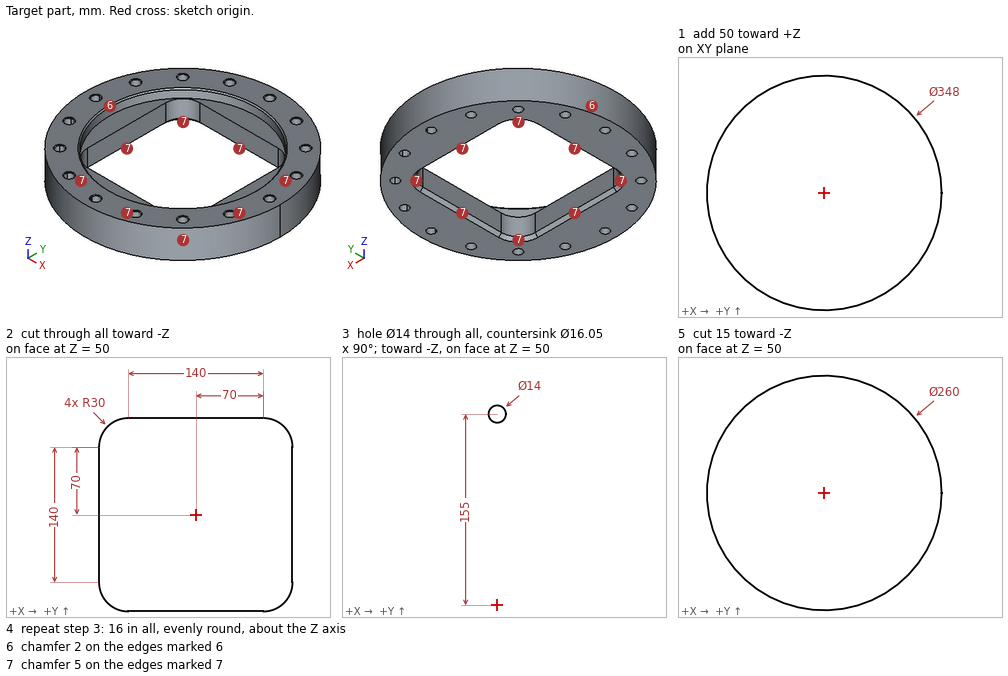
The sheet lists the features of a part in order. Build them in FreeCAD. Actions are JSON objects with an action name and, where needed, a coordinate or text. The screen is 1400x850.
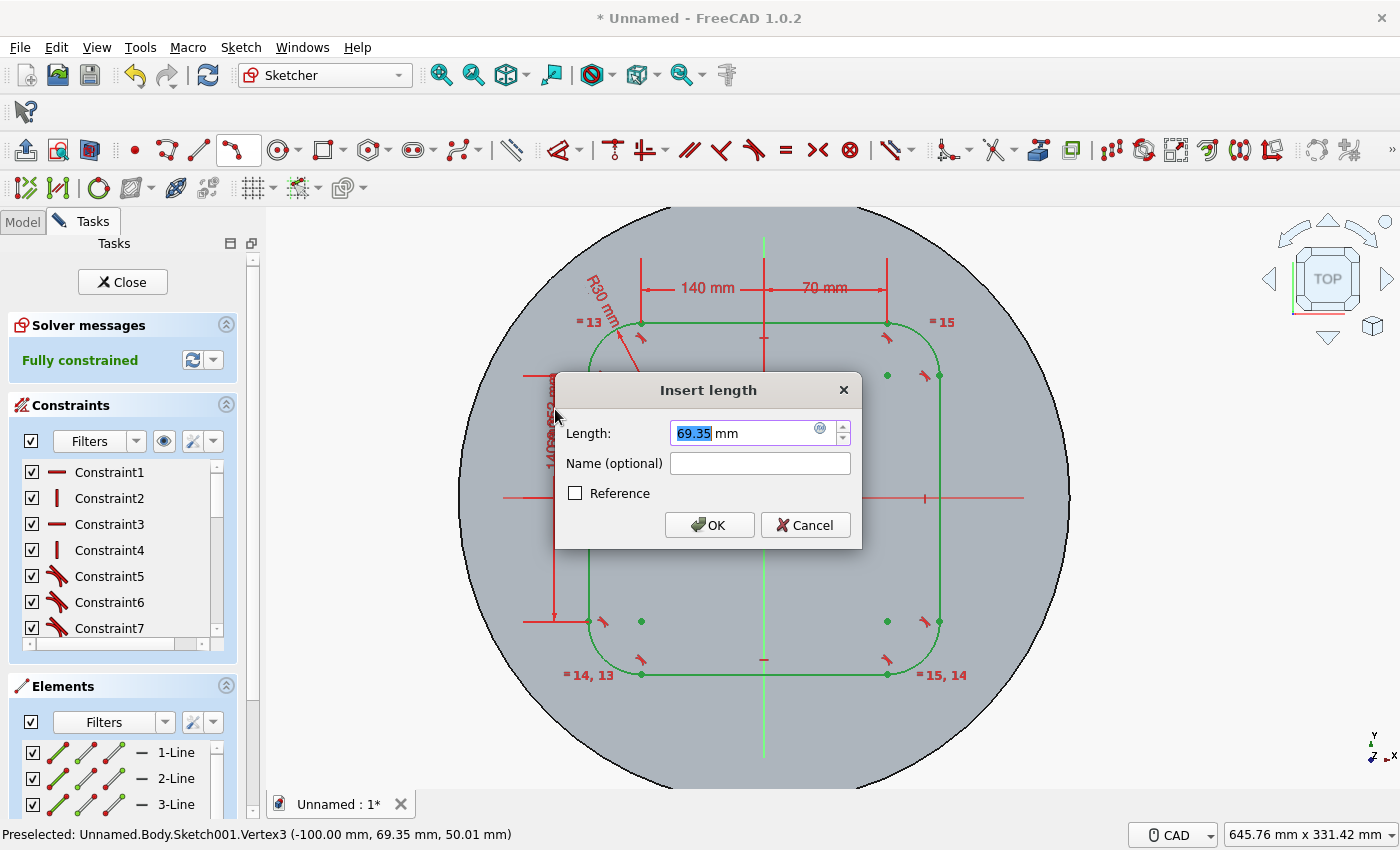
{"action": "type", "text": "70"}
{"action": "key", "text": "Return"}
{"action": "key", "text": "Escape"}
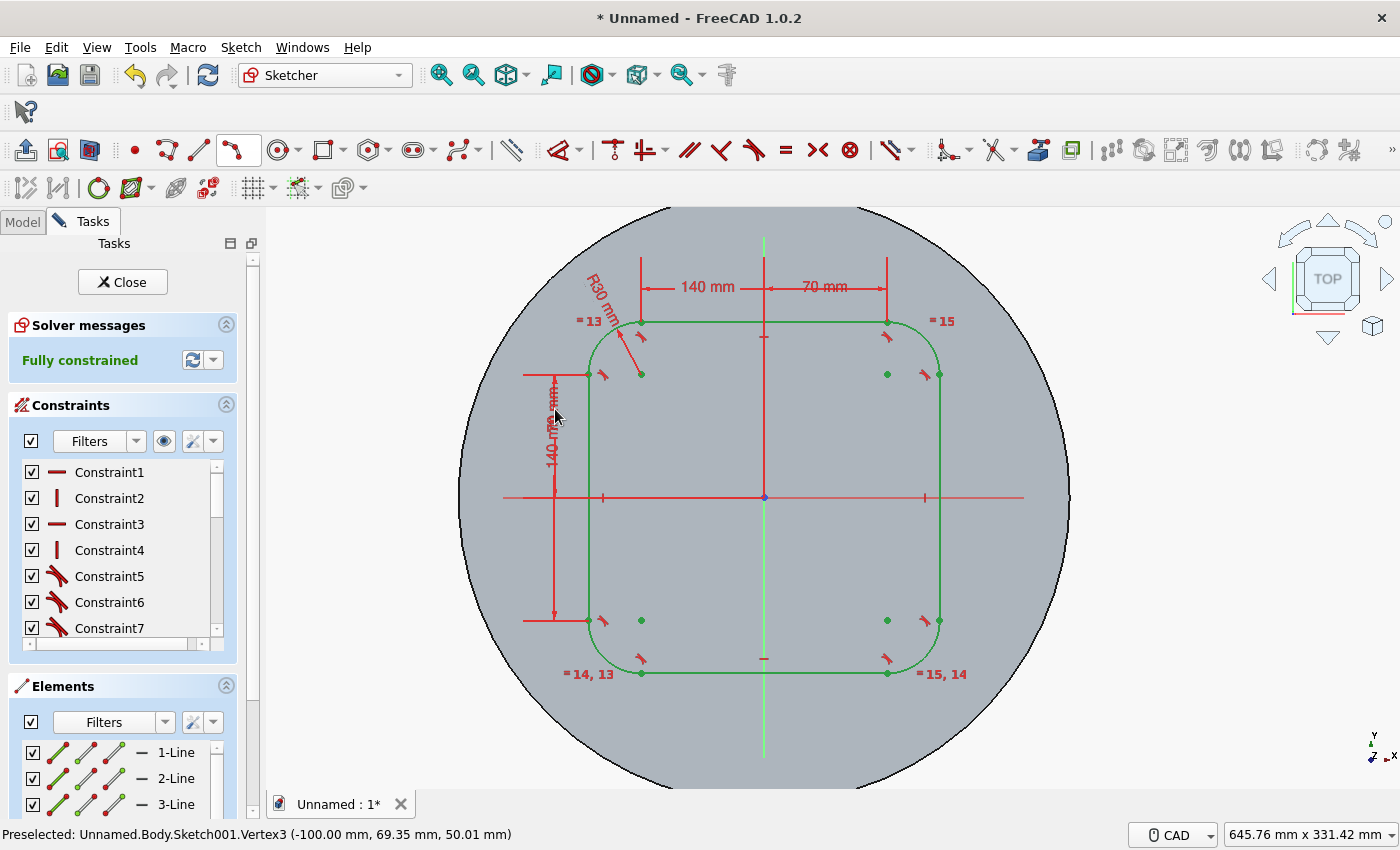
{"action": "left_click", "coordinate": [123, 282]}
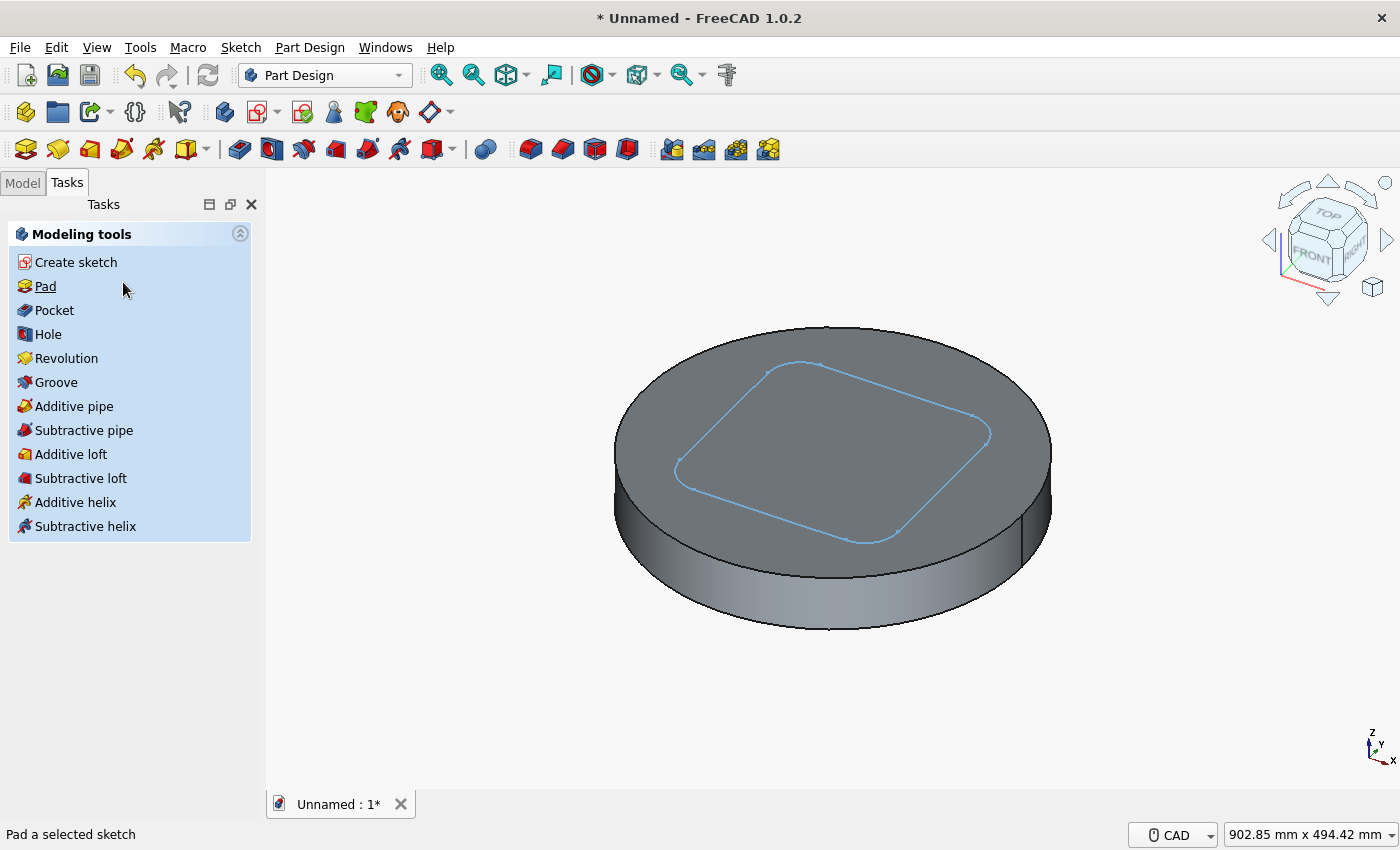
{"action": "left_click", "coordinate": [240, 150]}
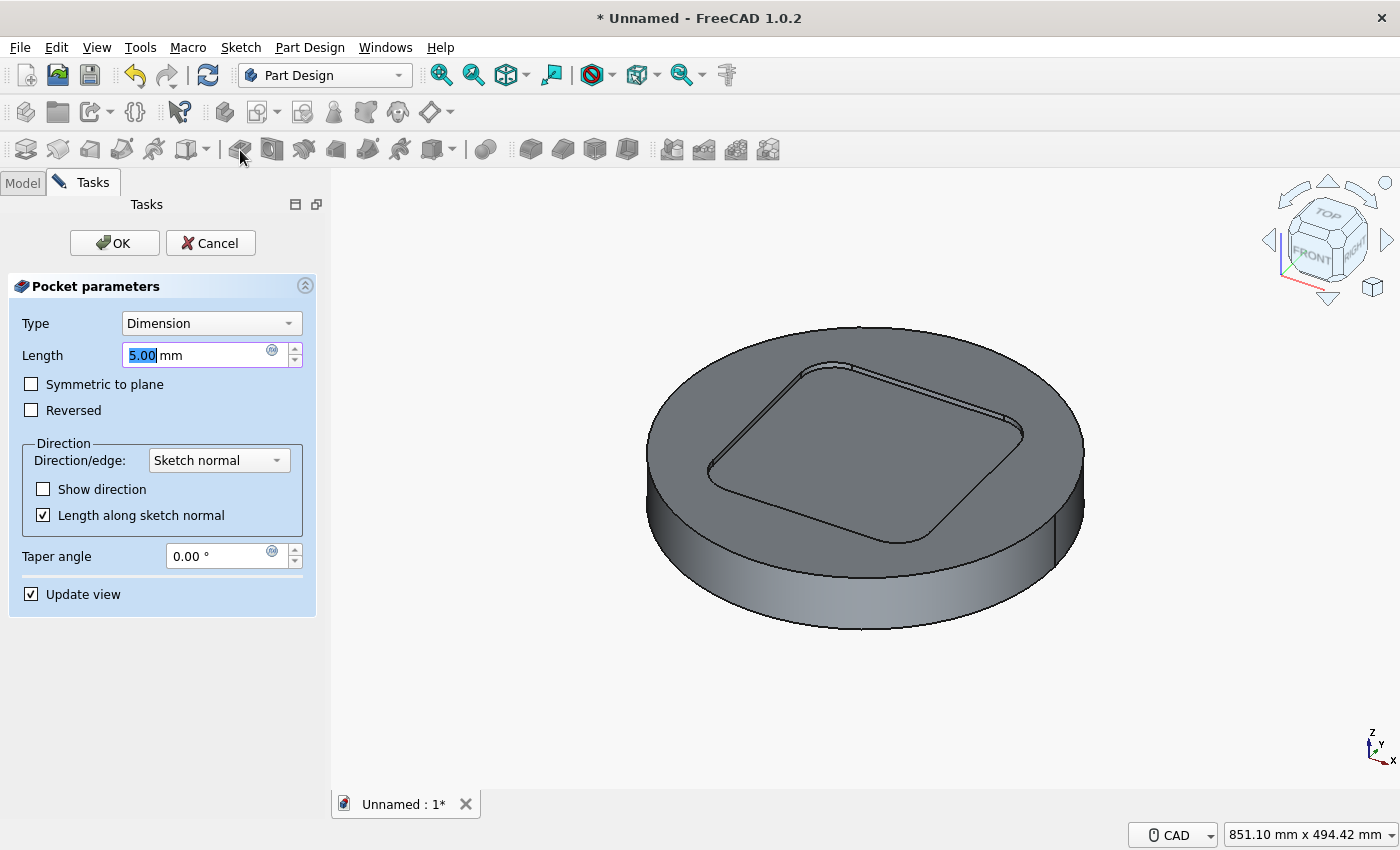
{"action": "left_click", "coordinate": [212, 324]}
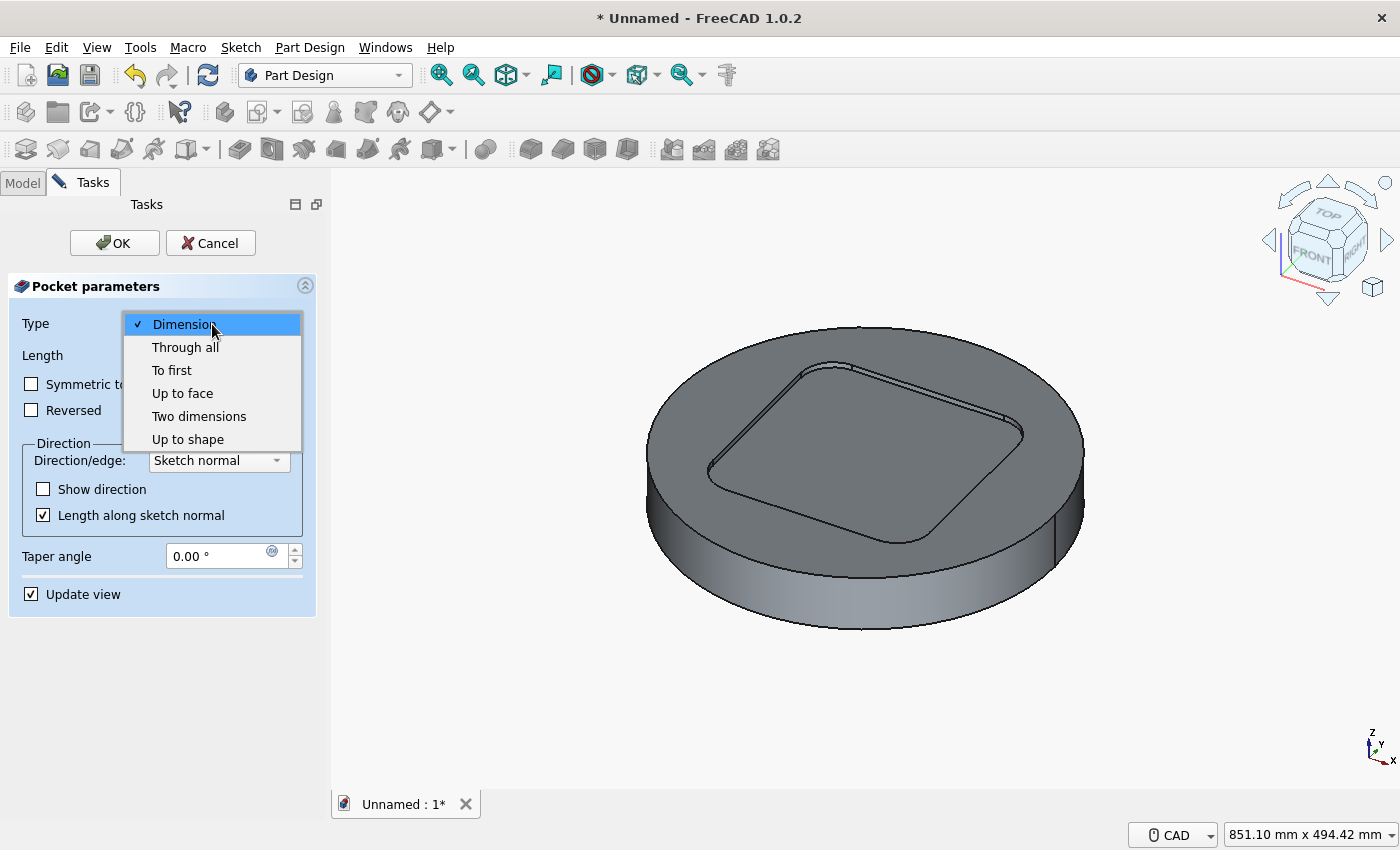
{"action": "left_click", "coordinate": [212, 348]}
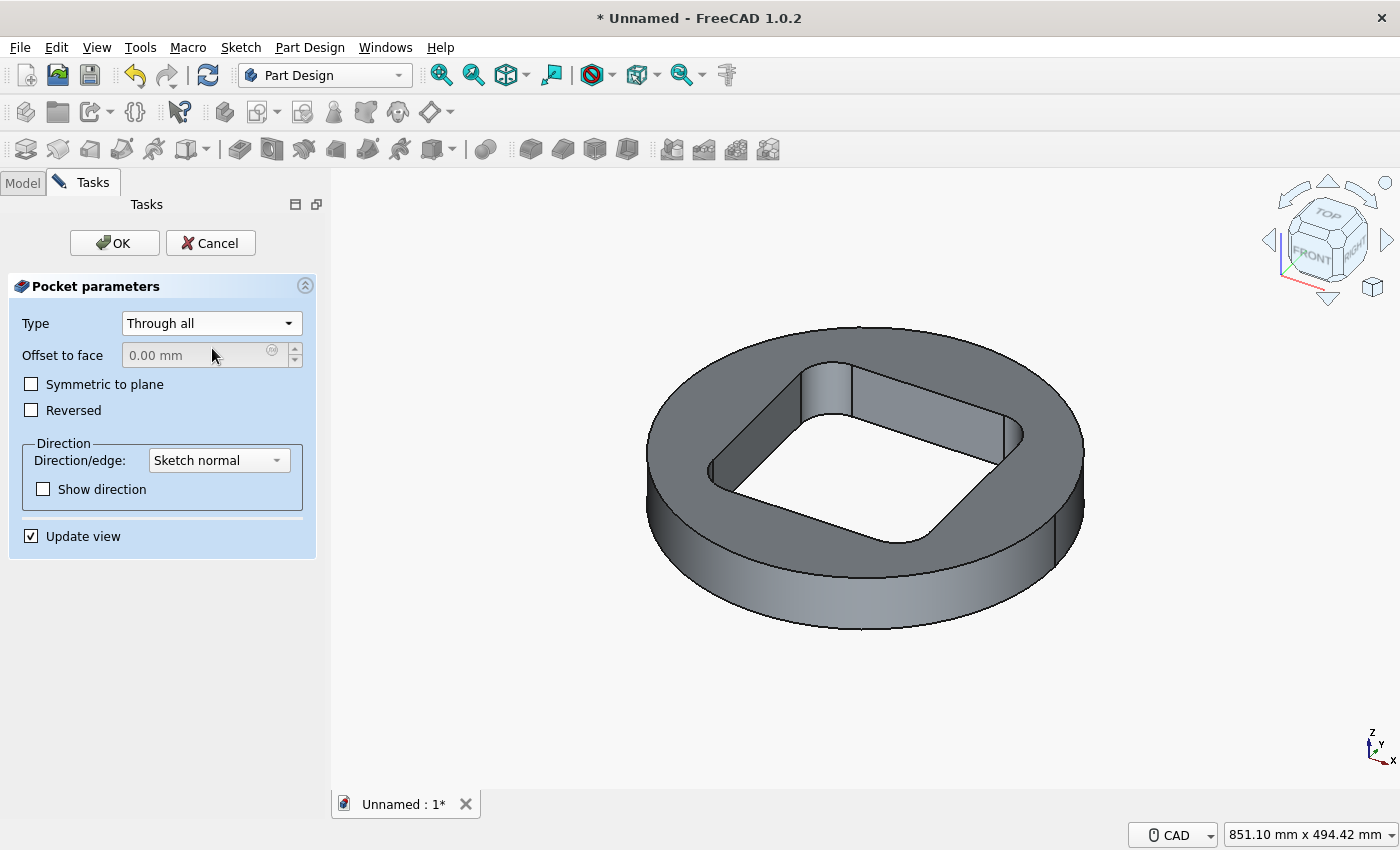
{"action": "left_click", "coordinate": [115, 243]}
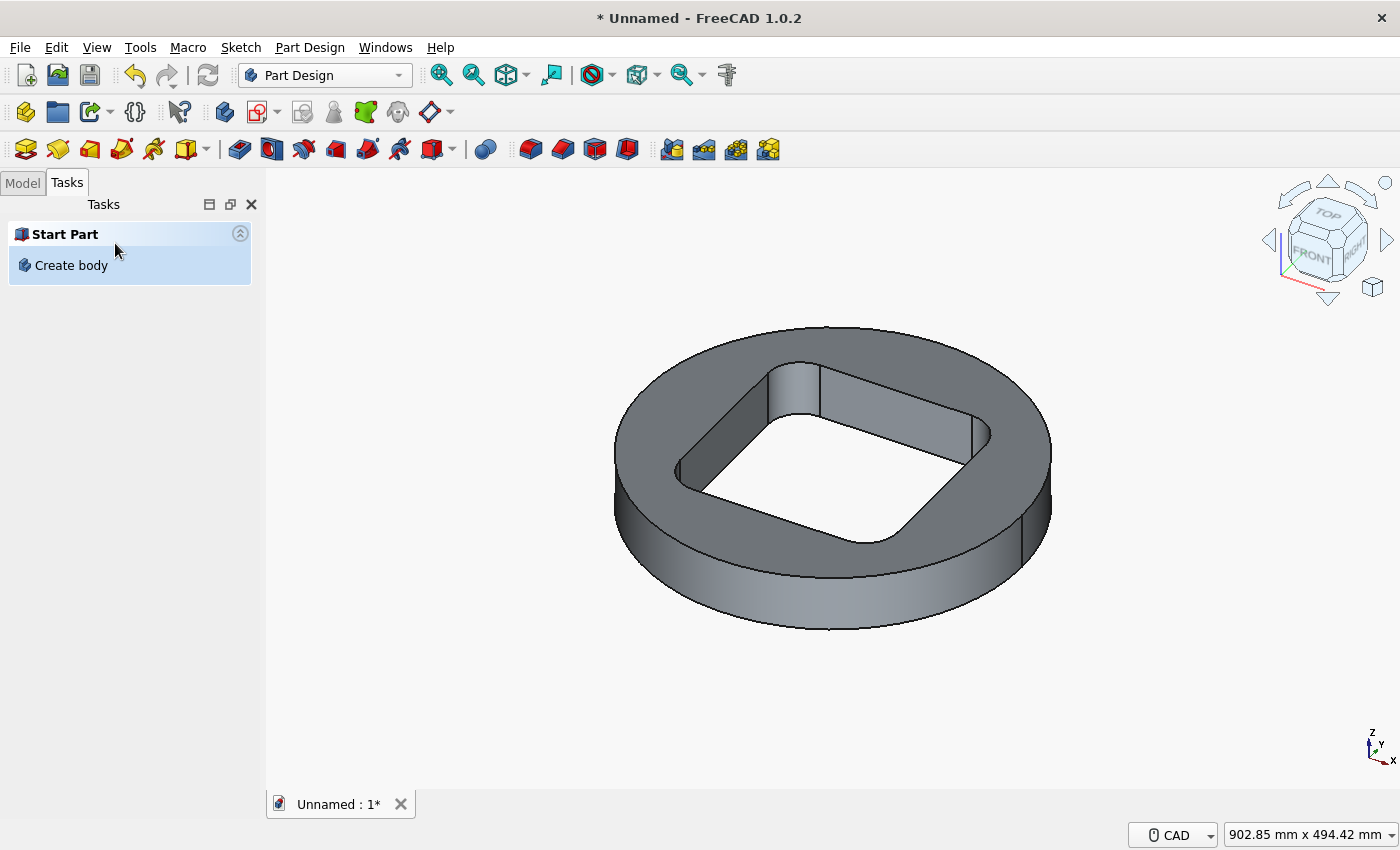
{"action": "left_click", "coordinate": [739, 545]}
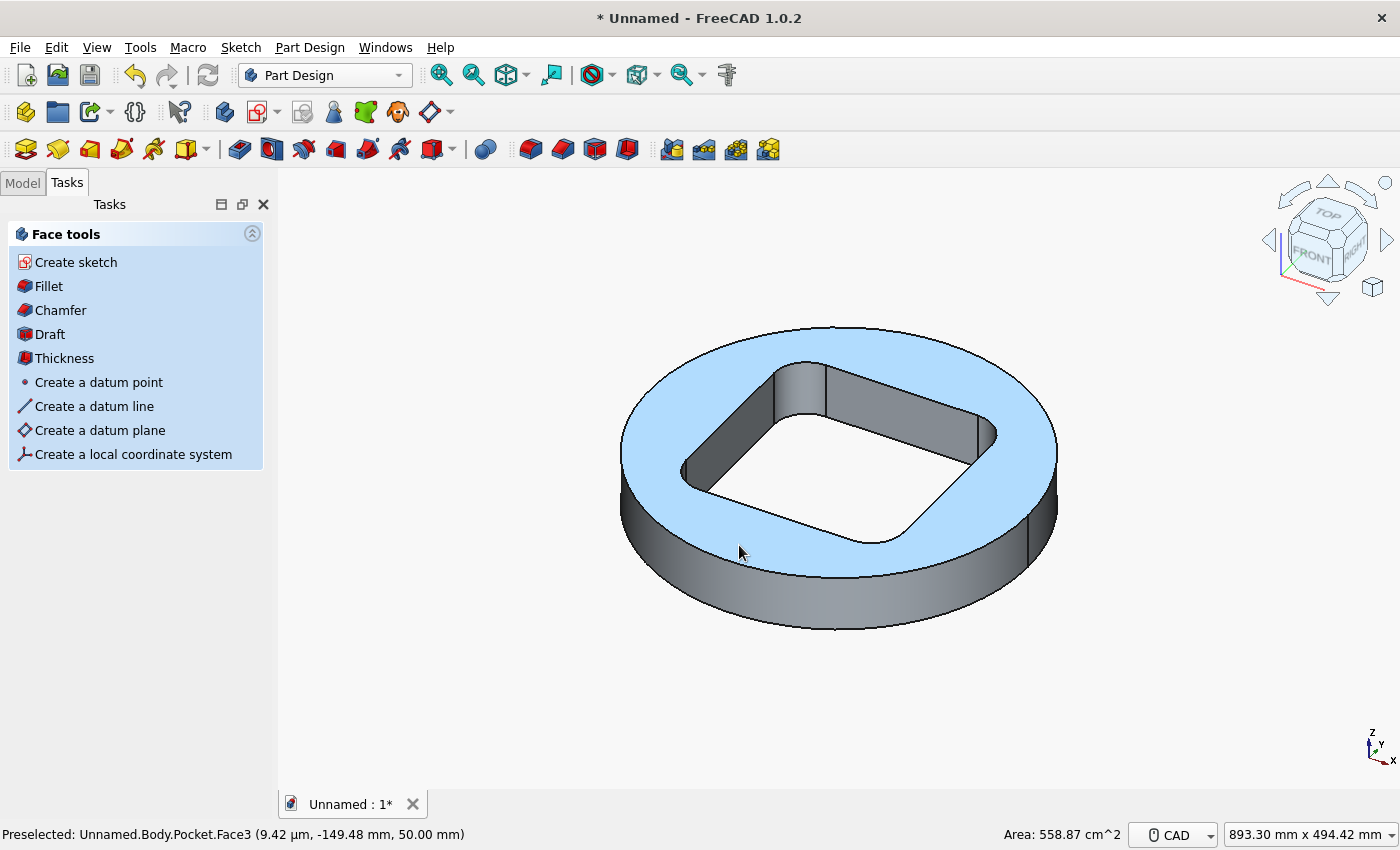
{"action": "left_click", "coordinate": [258, 112]}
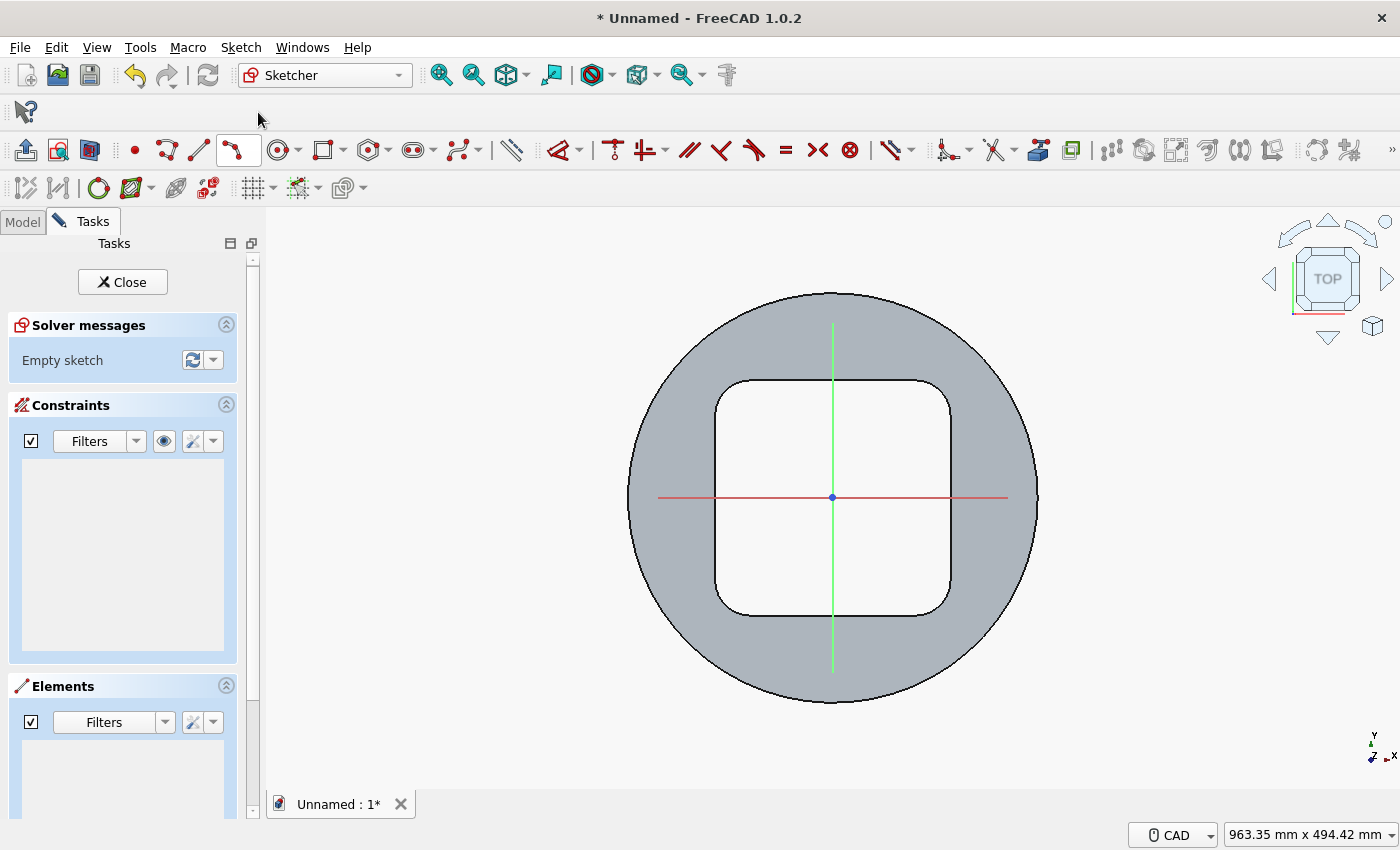
{"action": "scroll", "coordinate": [836, 306], "scroll_direction": "up", "scroll_amount": 15}